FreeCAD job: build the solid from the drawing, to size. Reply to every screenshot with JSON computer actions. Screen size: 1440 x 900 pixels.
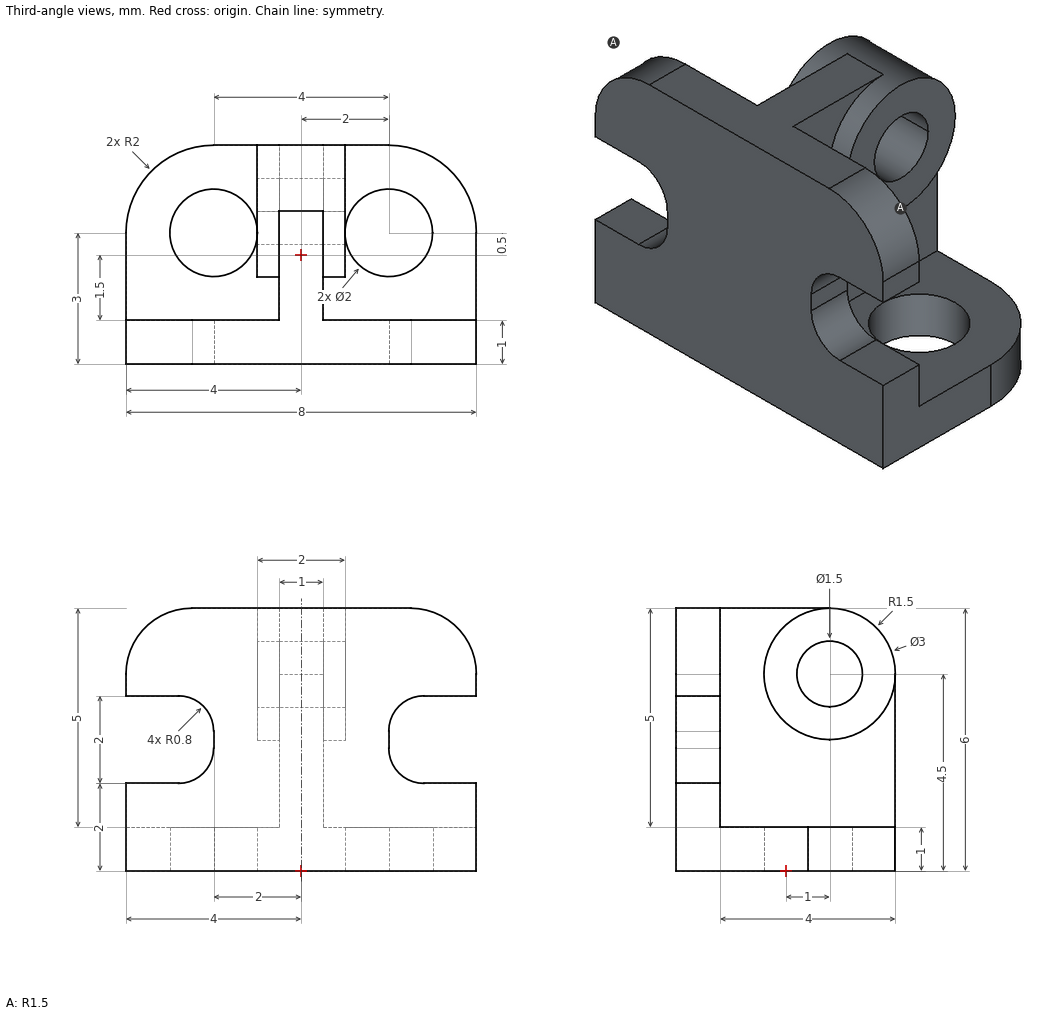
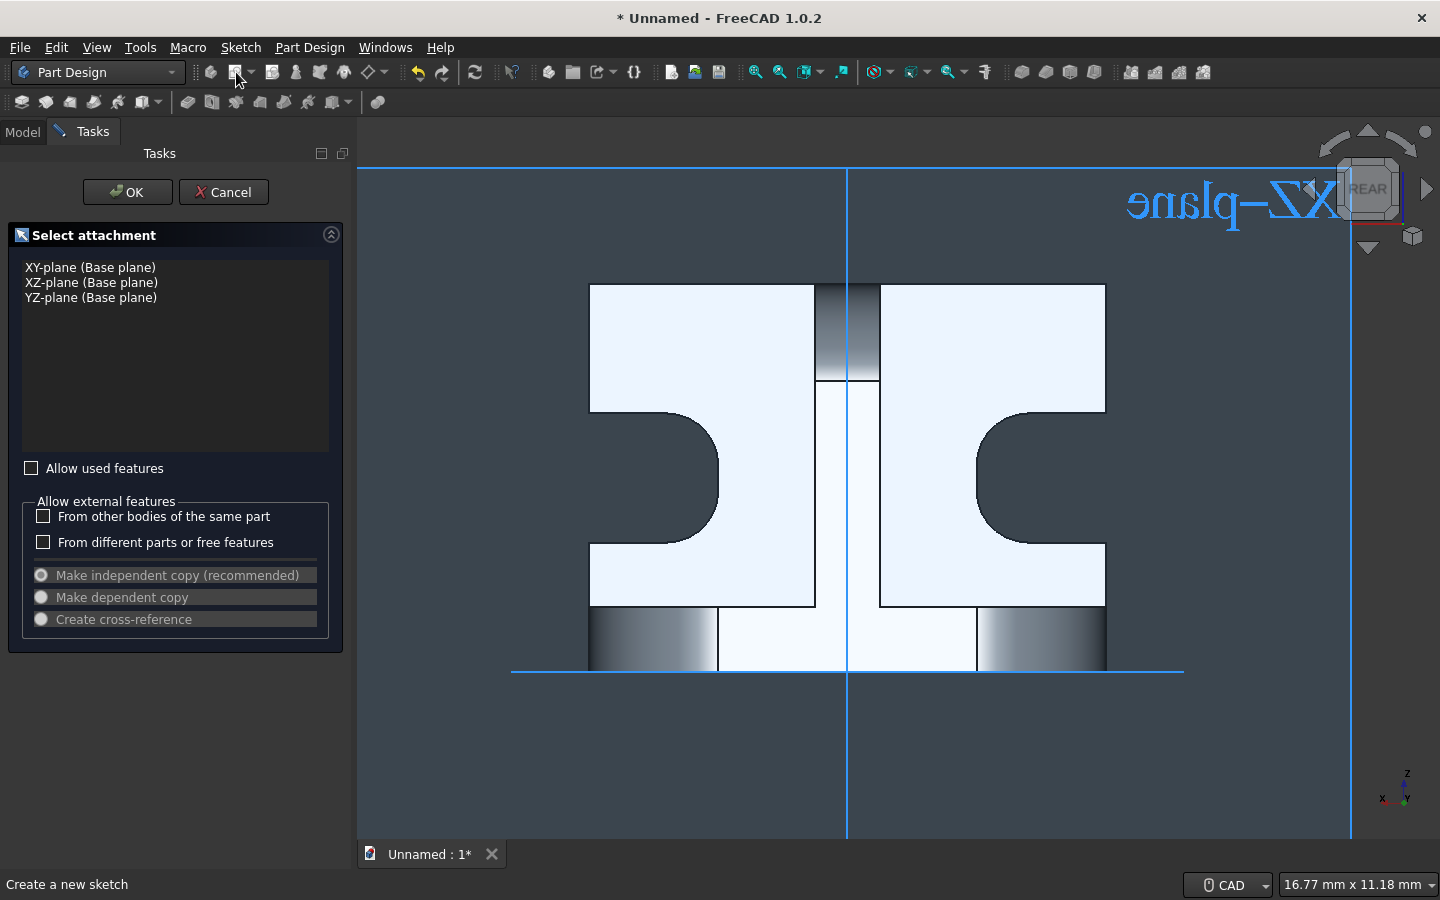
{"action": "left_click", "coordinate": [82, 298]}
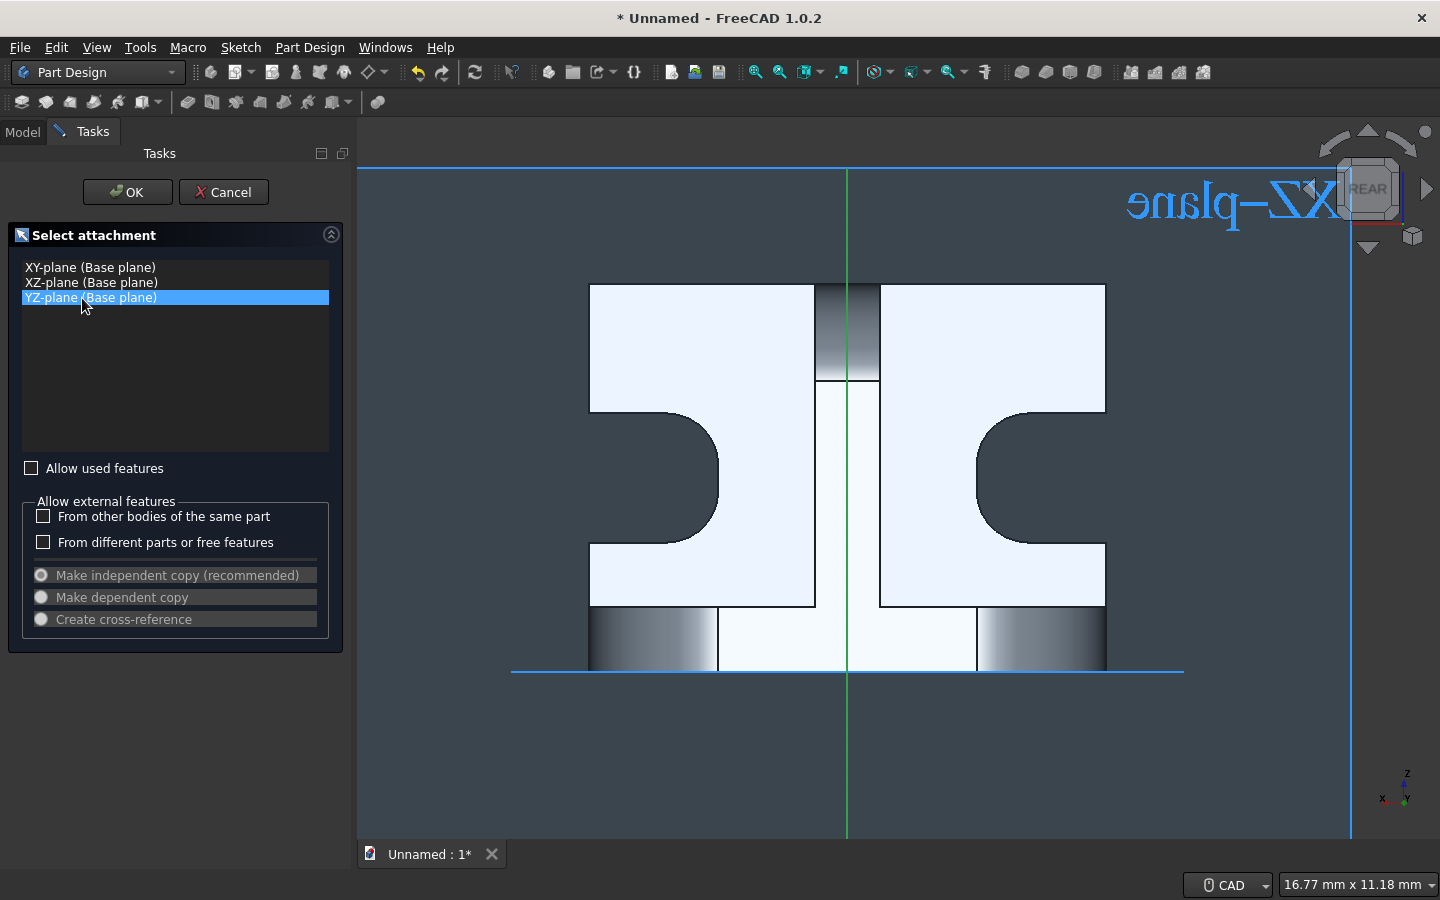
{"action": "left_click", "coordinate": [128, 192]}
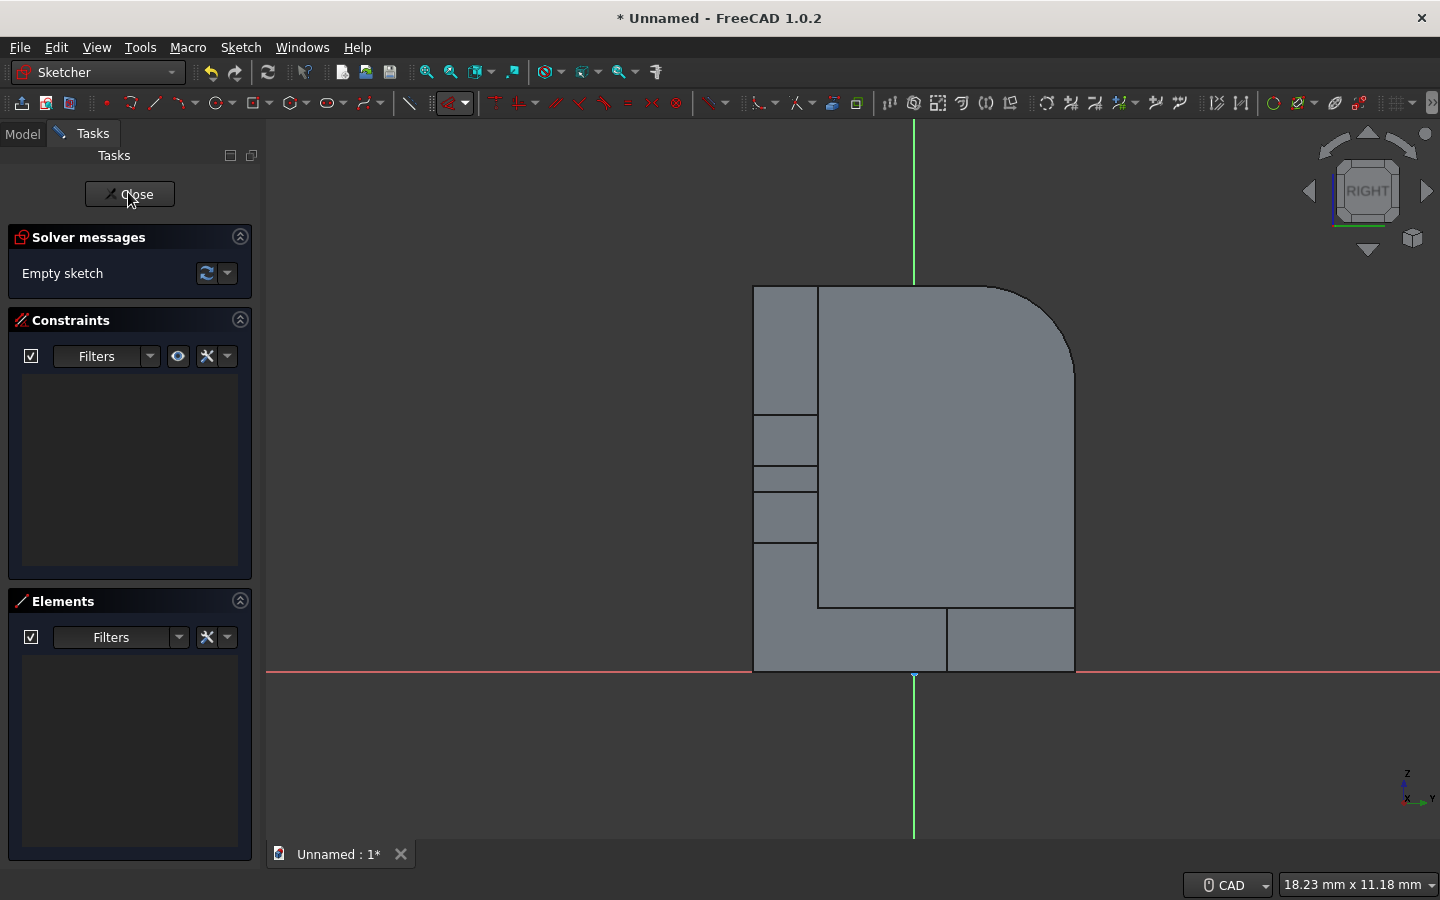
{"action": "left_click", "coordinate": [70, 104]}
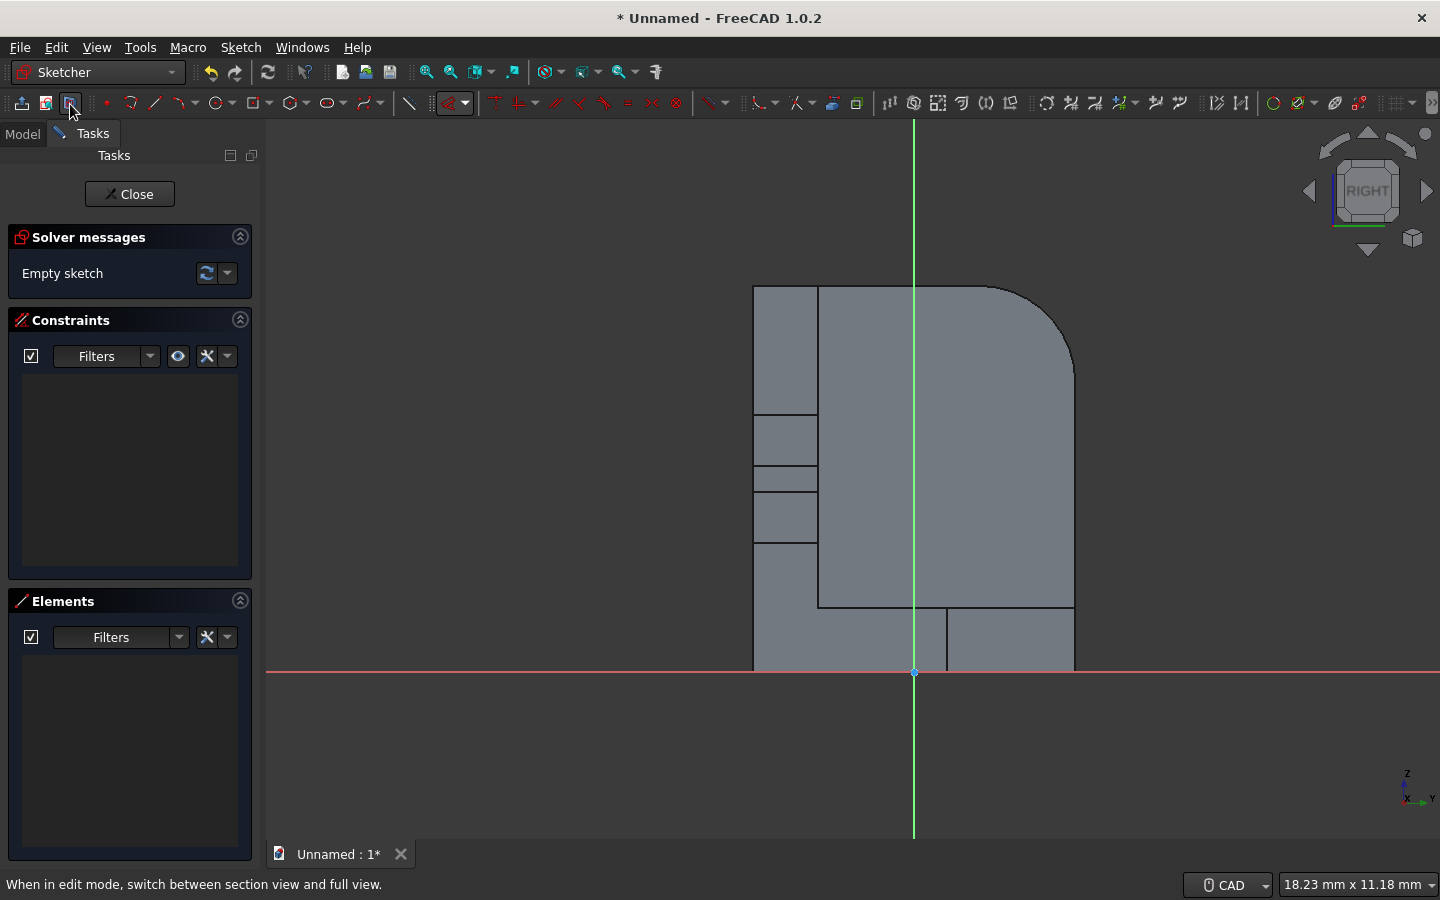
{"action": "left_click", "coordinate": [216, 104]}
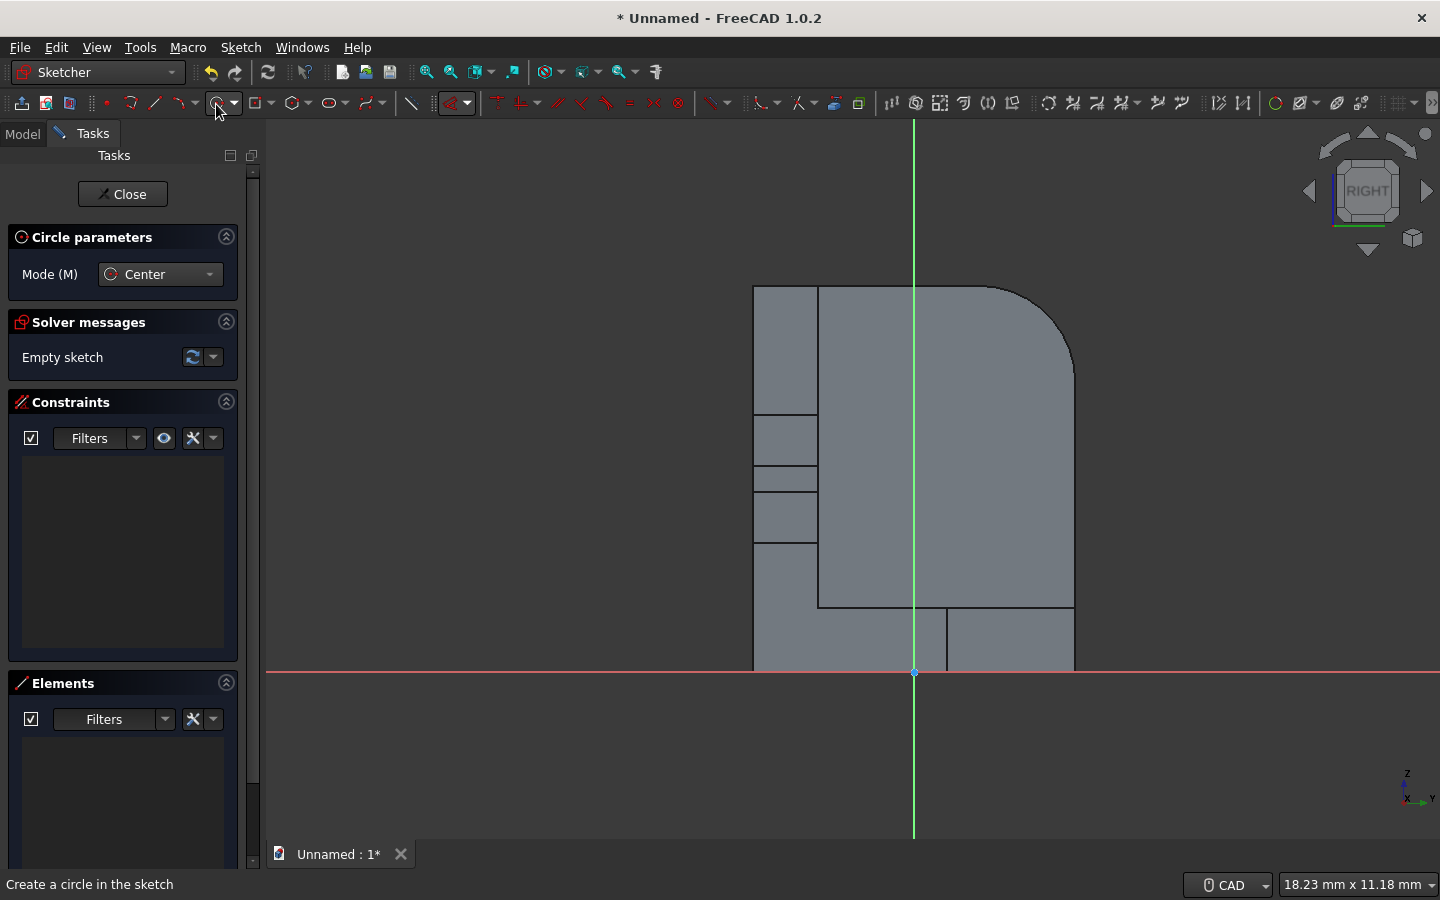
{"action": "left_click", "coordinate": [979, 382]}
{"action": "mouse_move", "coordinate": [1047, 314]}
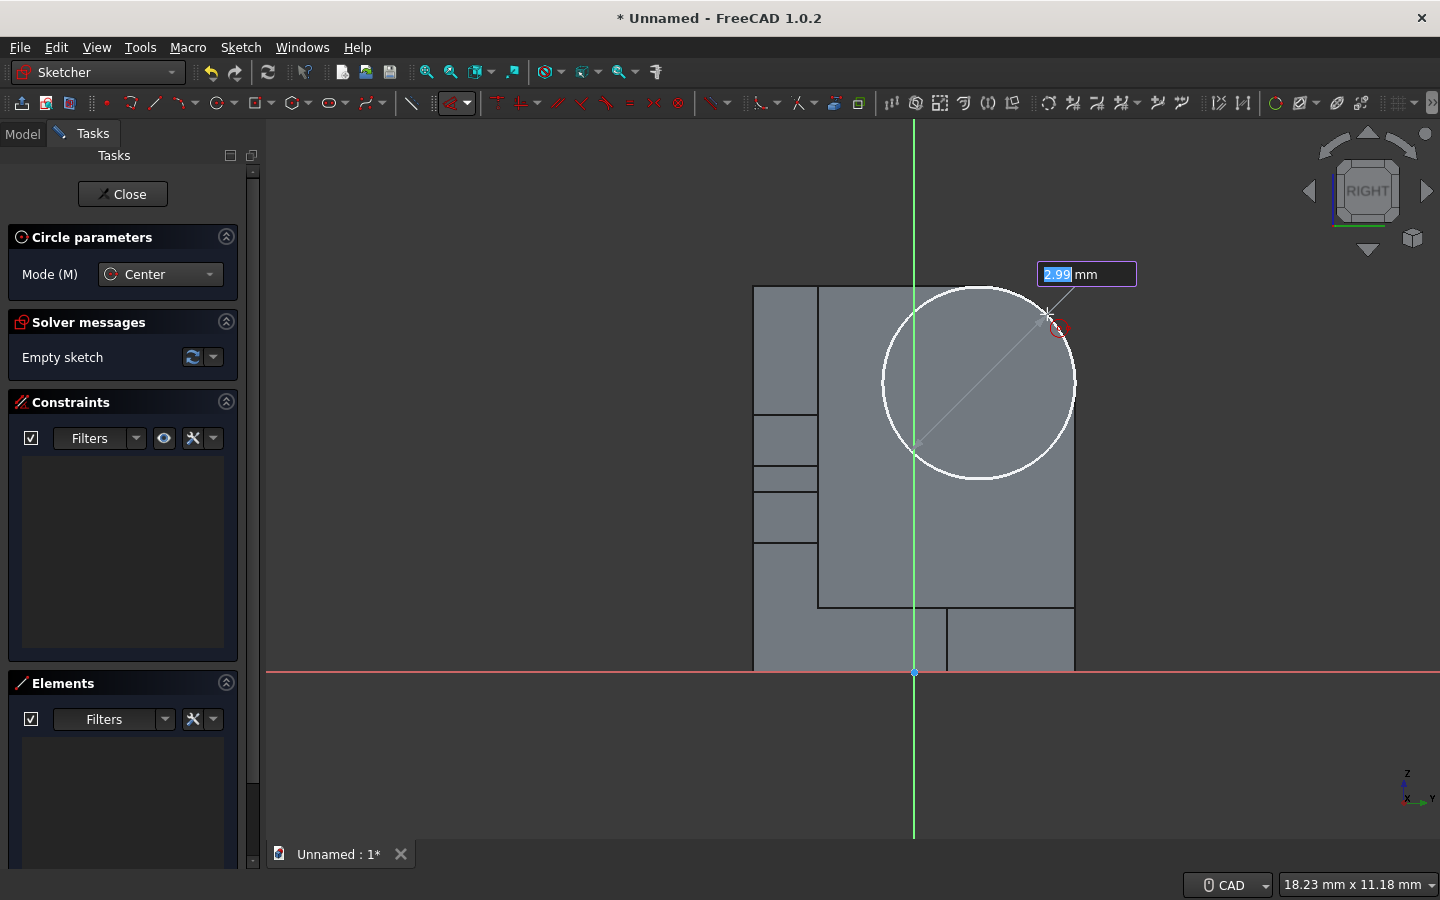
{"action": "type", "text": "3"}
{"action": "key", "text": "Return"}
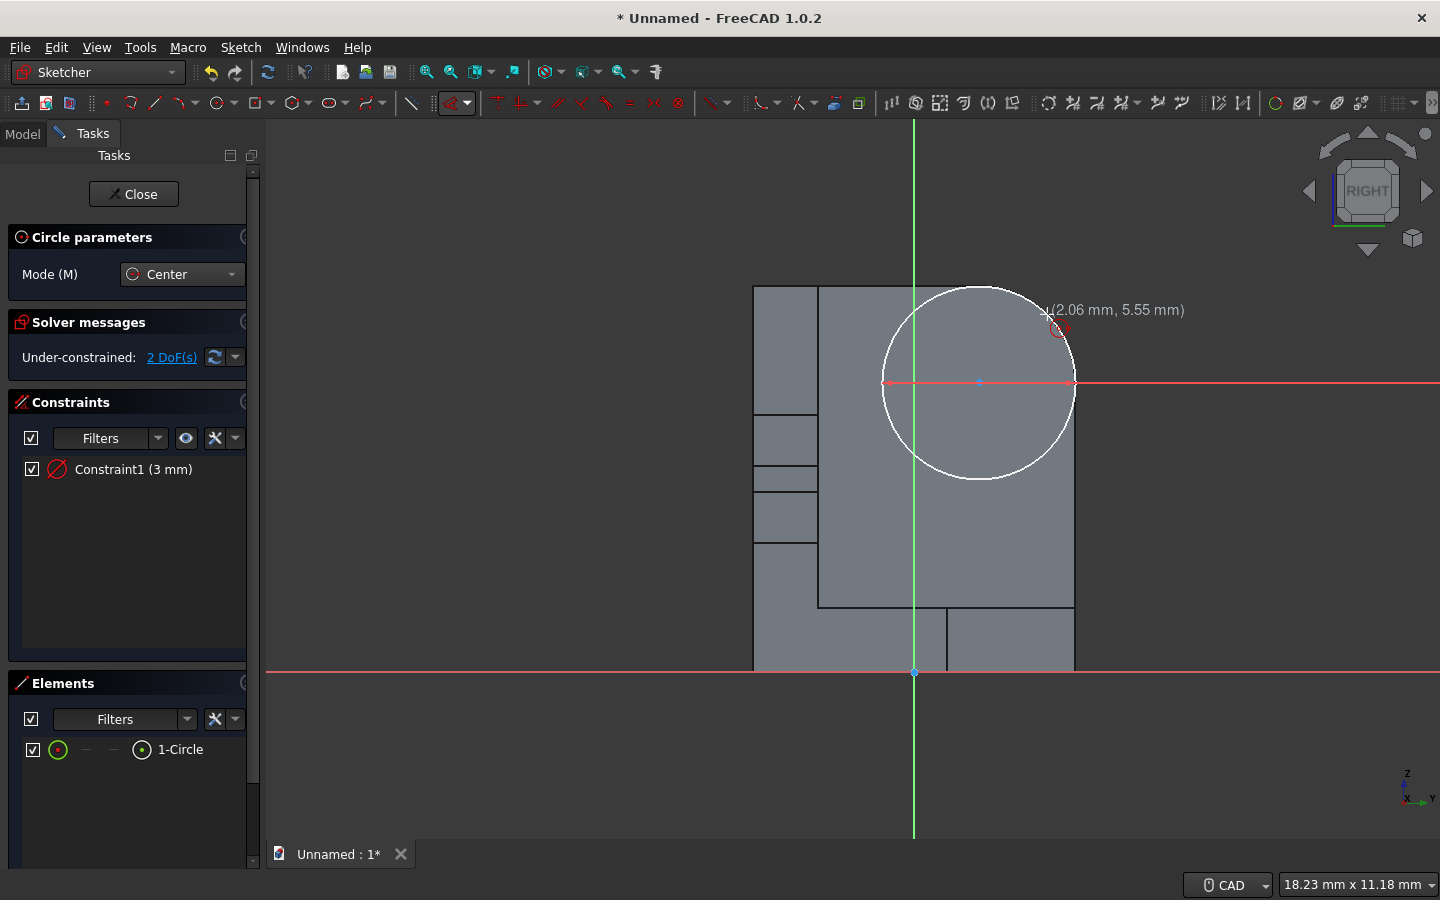
{"action": "left_click", "coordinate": [979, 383]}
{"action": "mouse_move", "coordinate": [1013, 348]}